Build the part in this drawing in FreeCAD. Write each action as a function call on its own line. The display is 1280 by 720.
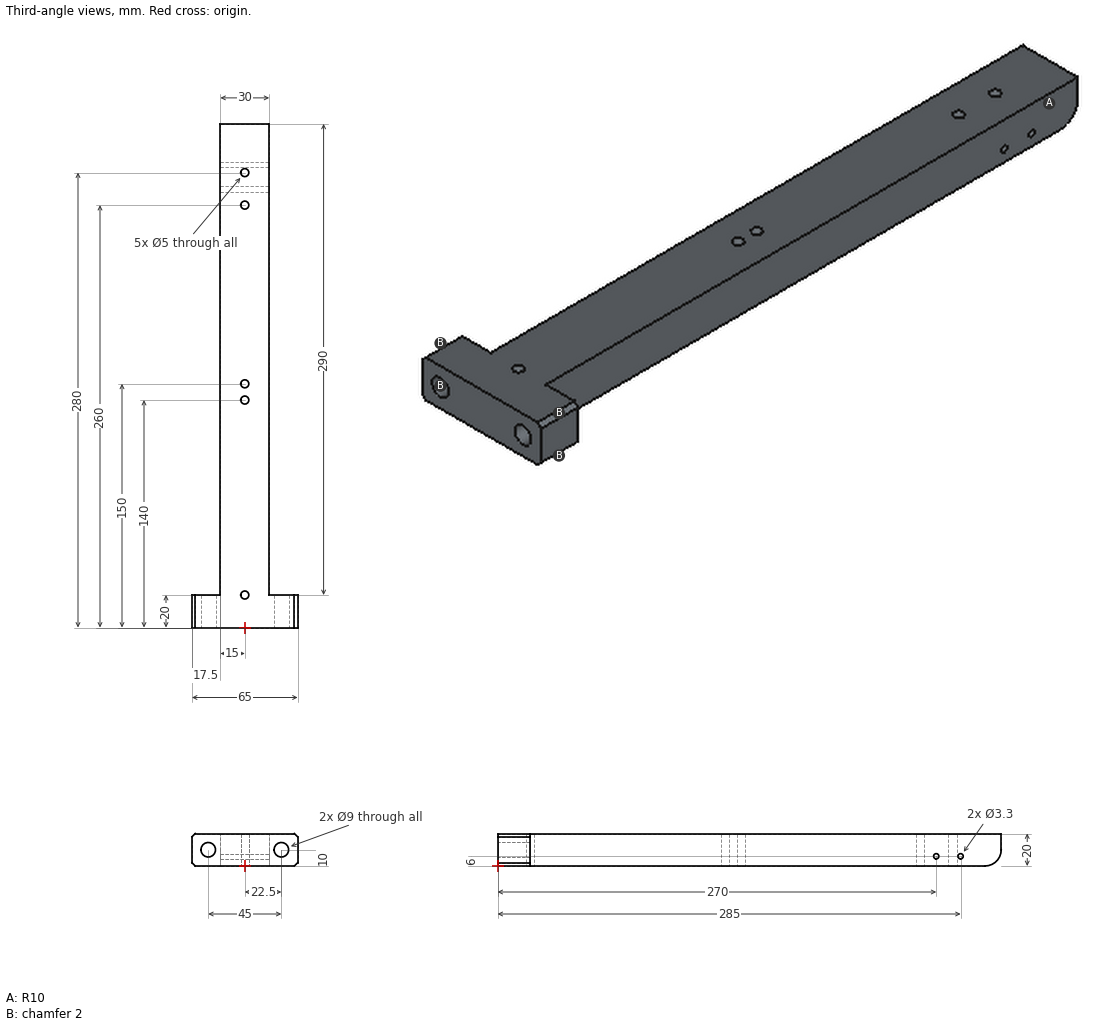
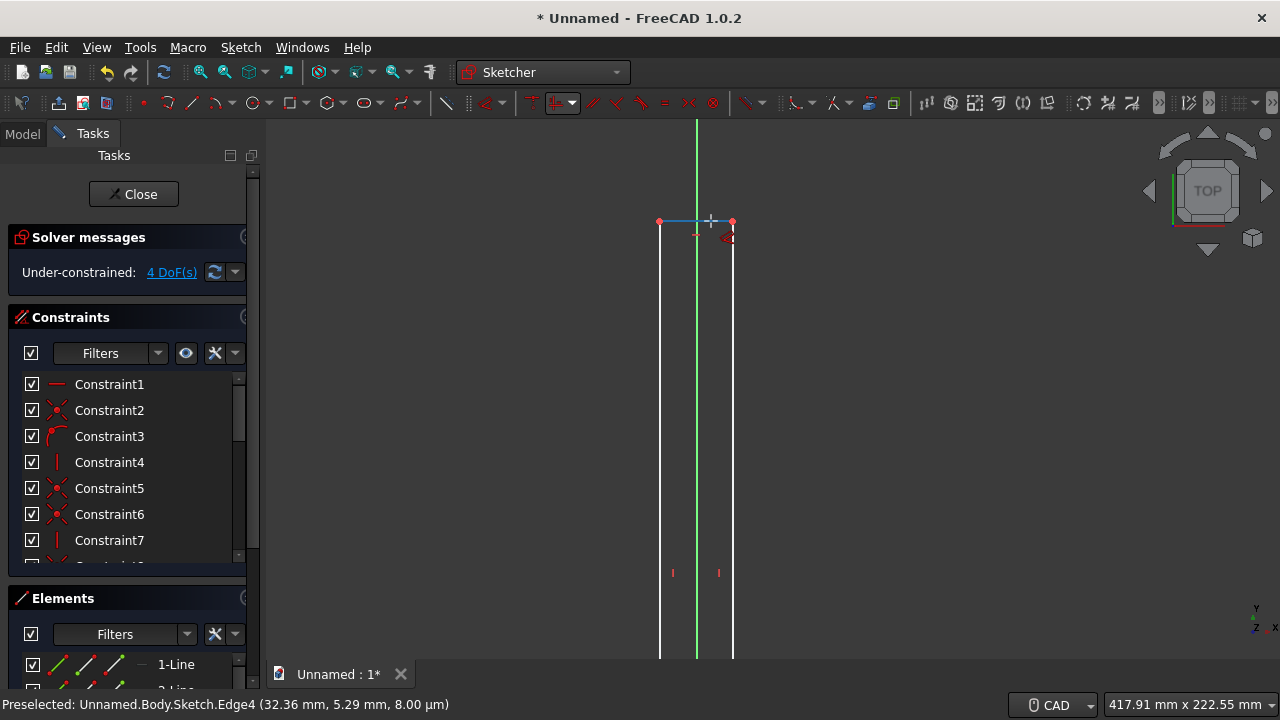
click(711, 221)
click(679, 187)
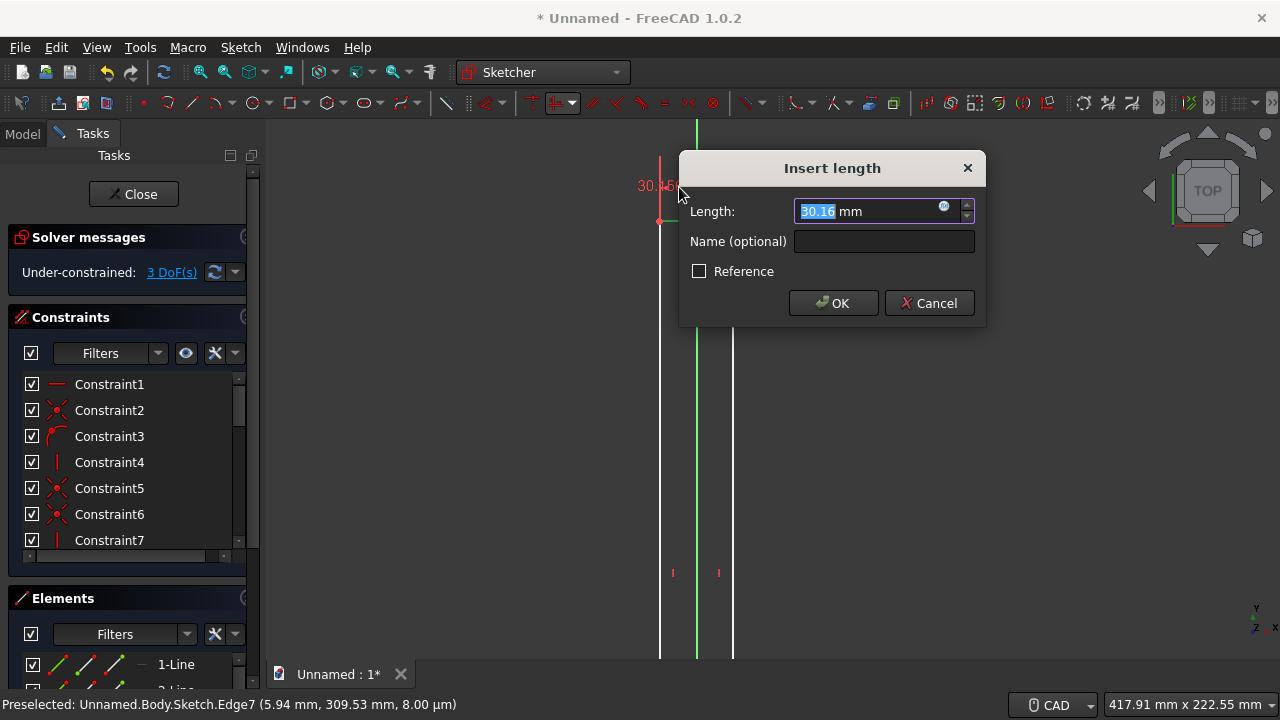
text(30)
key(Return)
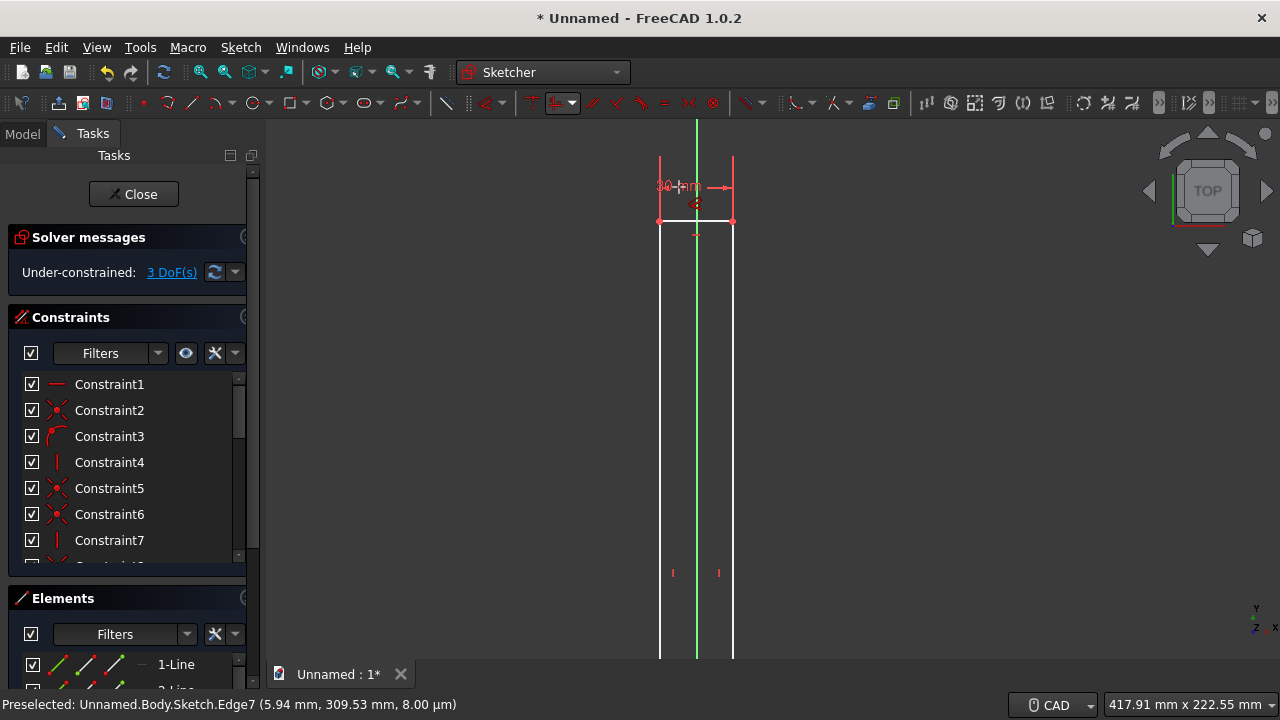
click(733, 432)
click(767, 426)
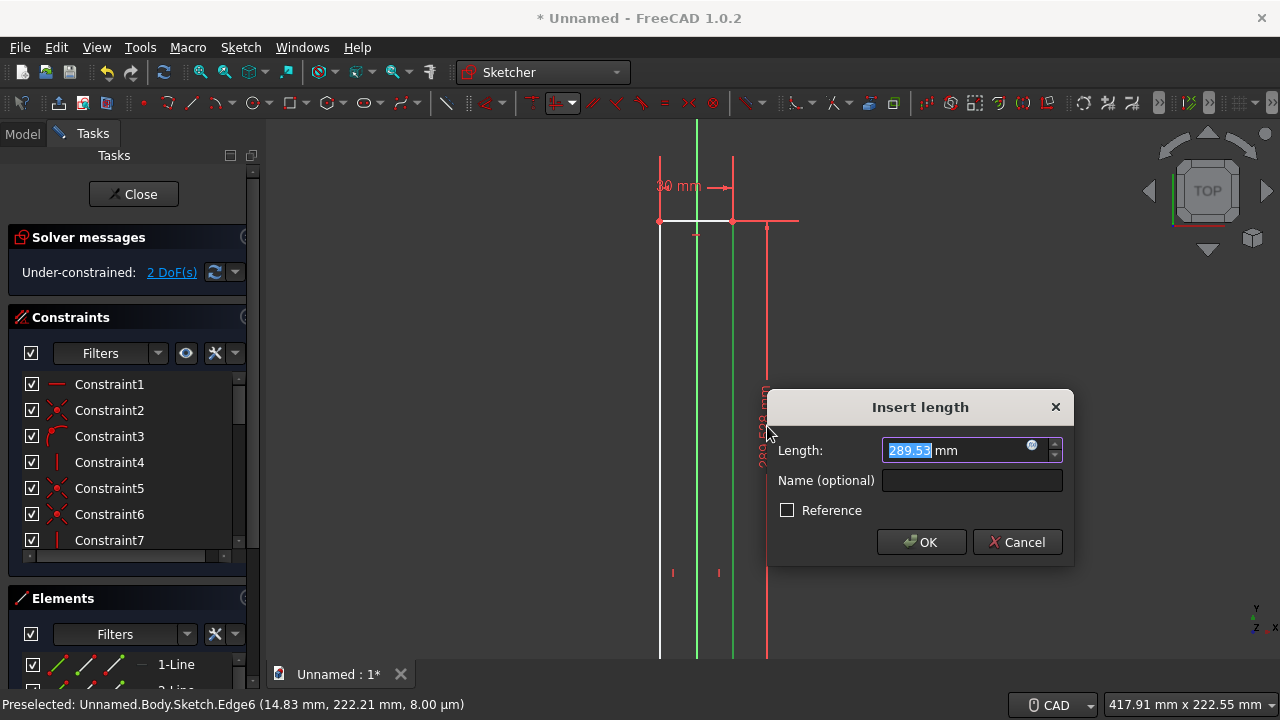
text(290)
key(Return)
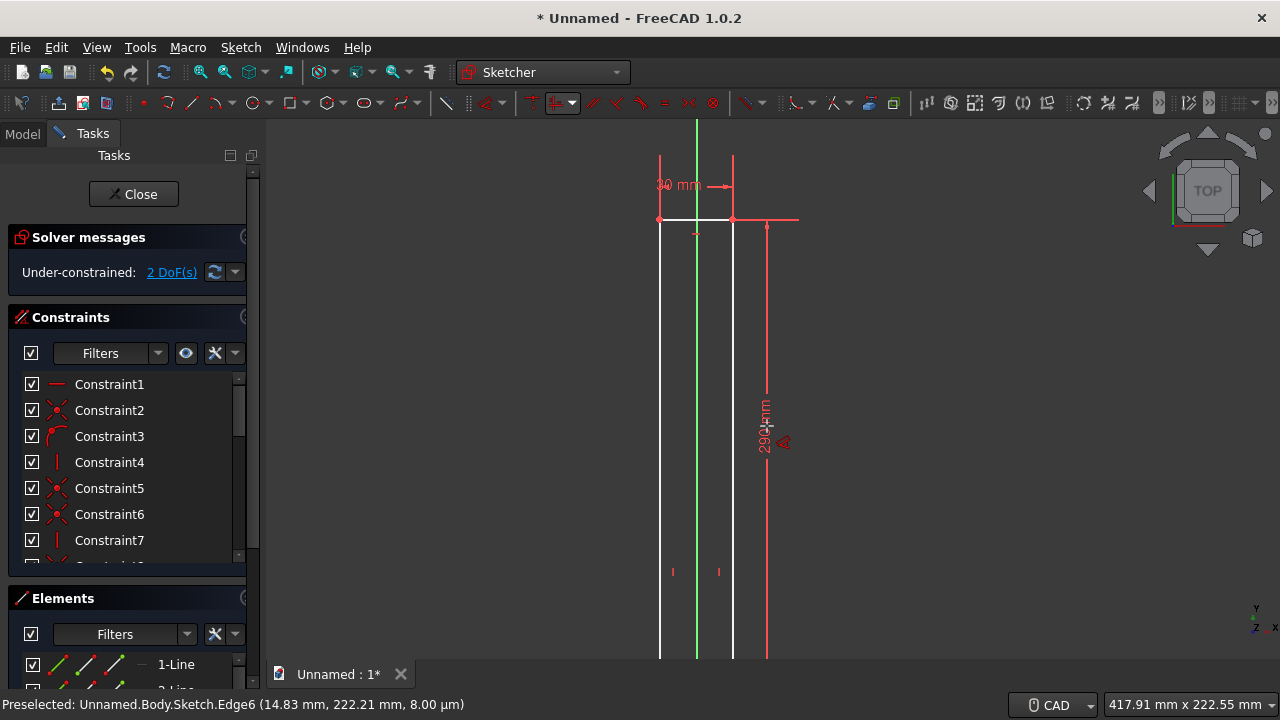
scroll(711, 220, down, 4)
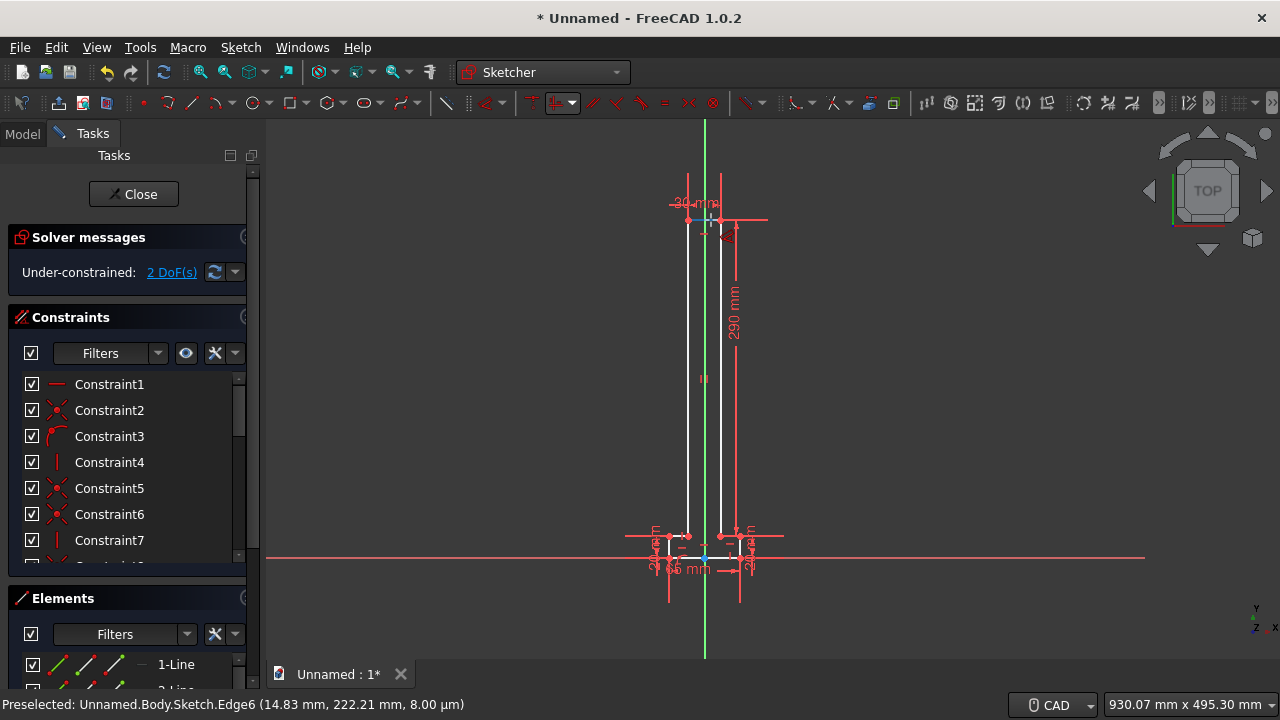
scroll(688, 536, up, 5)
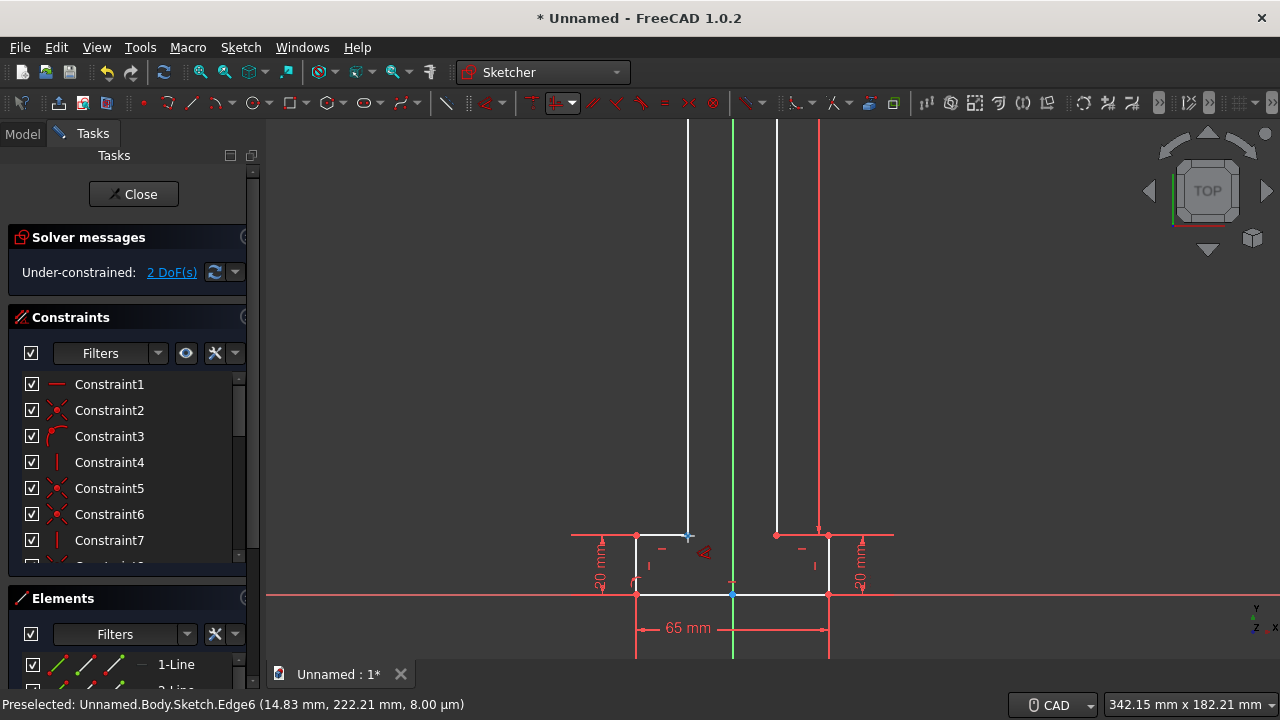
click(688, 535)
click(710, 501)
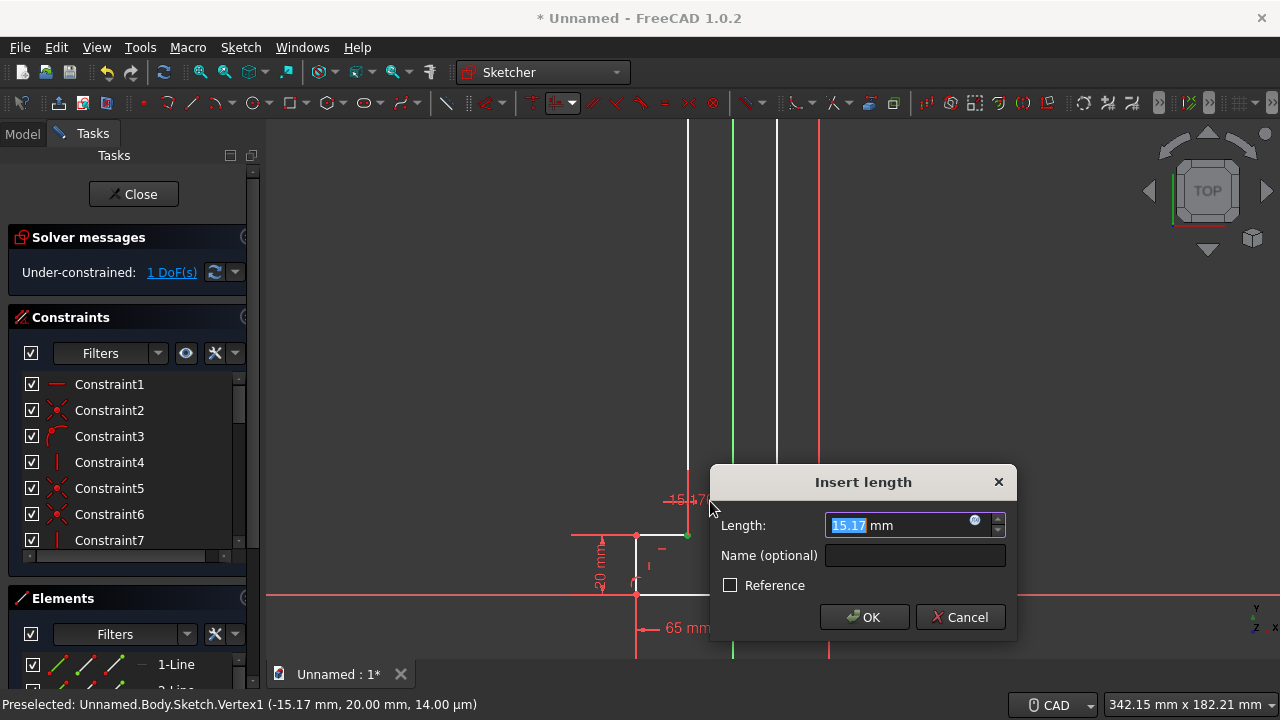
text(15)
key(Return)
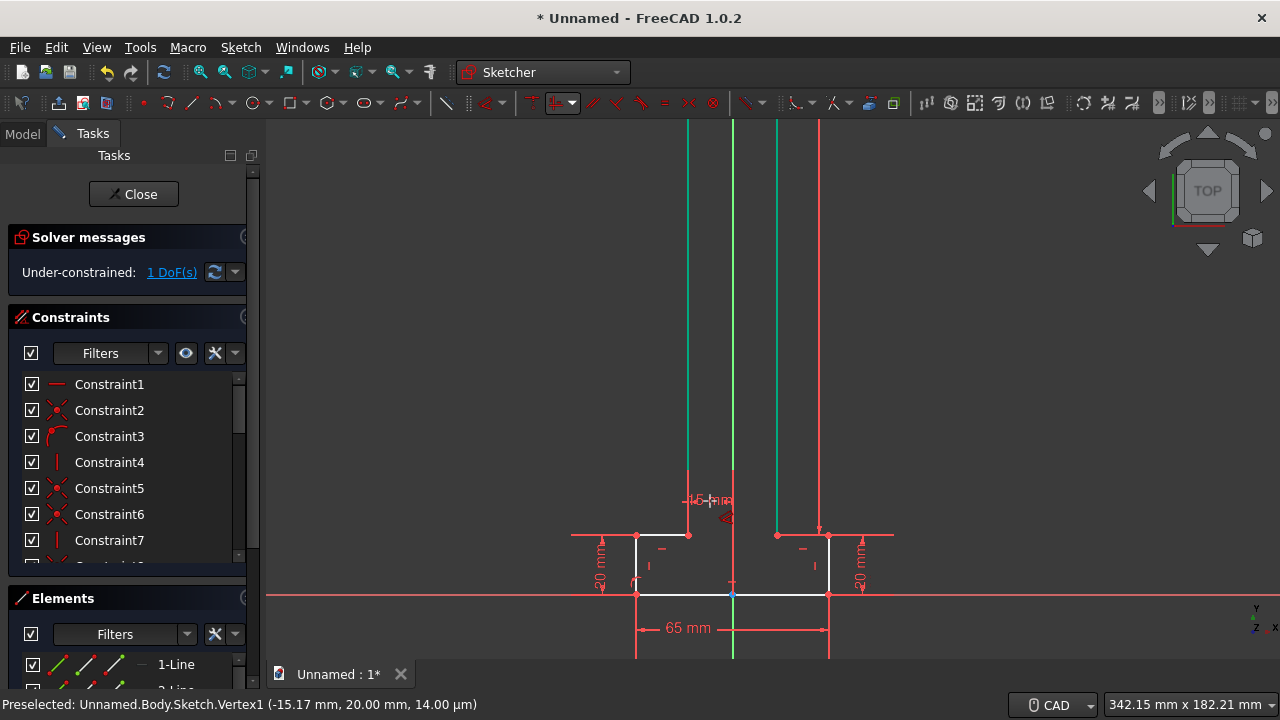
click(673, 535)
click(674, 569)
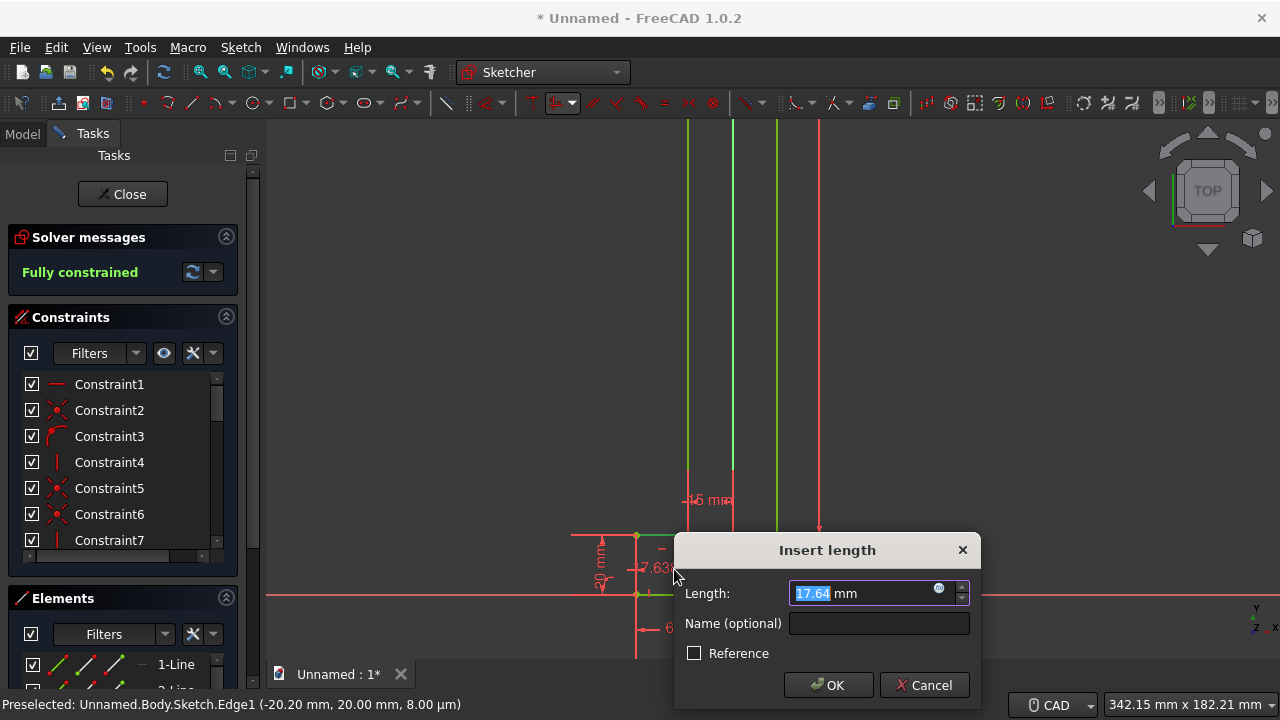
text(17.5)
key(Return)
key(Escape)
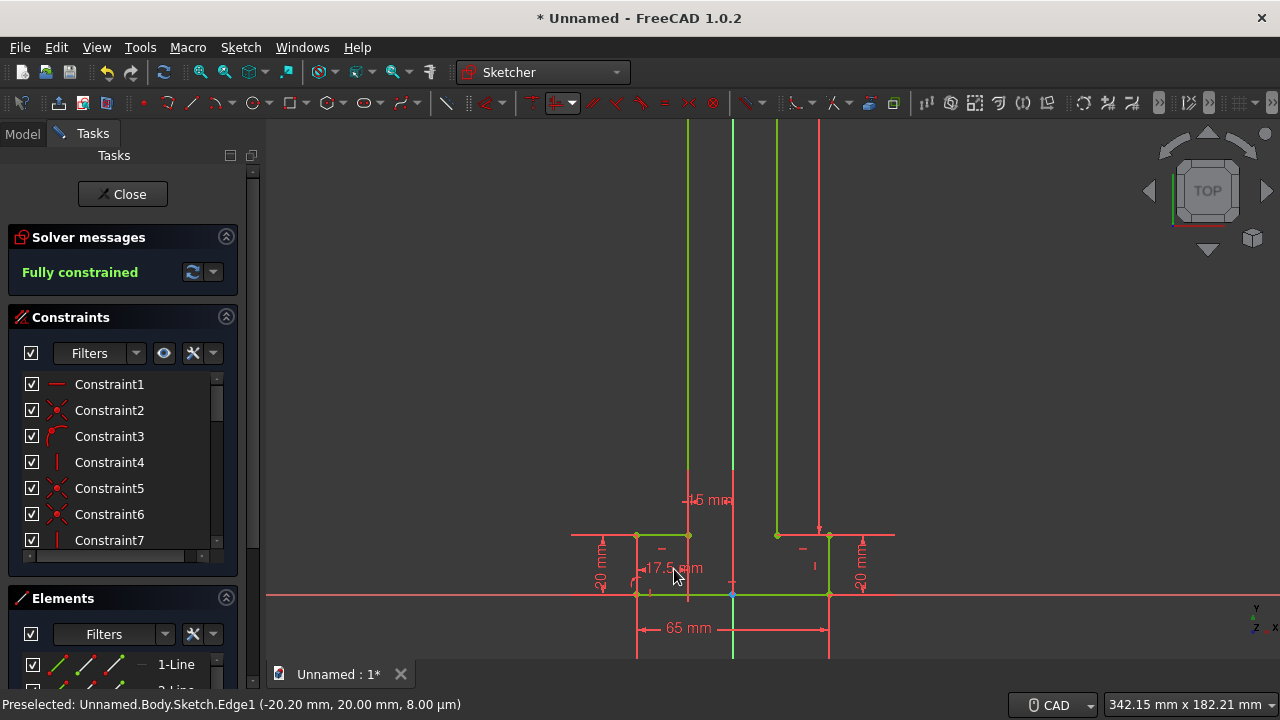
click(123, 194)